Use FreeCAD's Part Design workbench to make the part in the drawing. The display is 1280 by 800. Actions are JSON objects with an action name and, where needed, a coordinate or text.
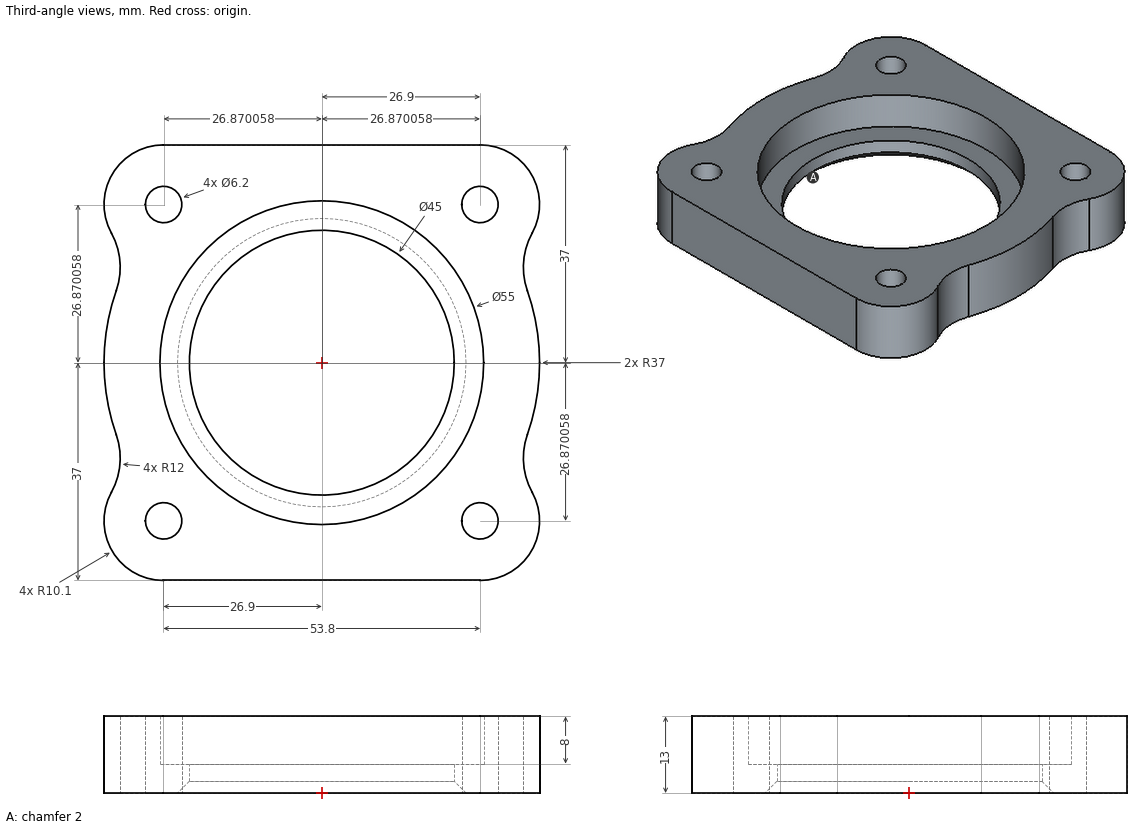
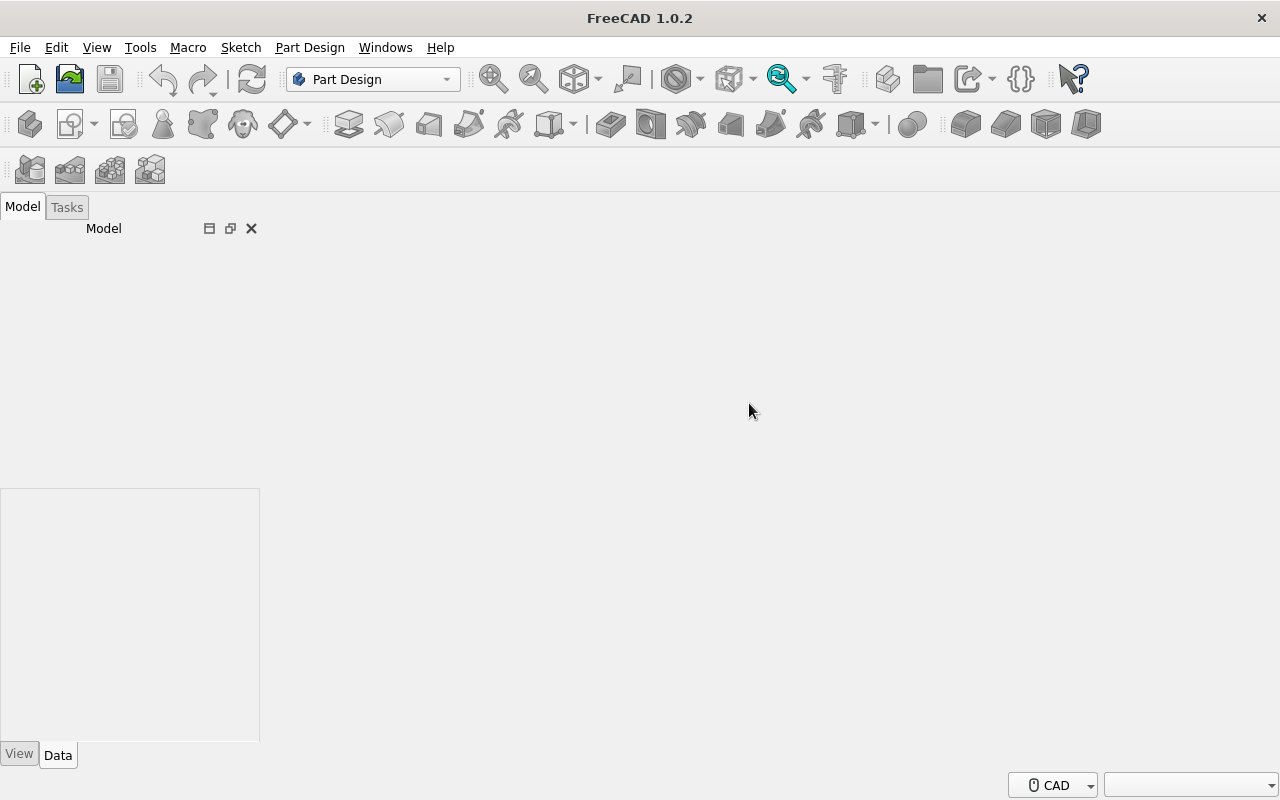
{"action": "key", "text": "ctrl+n"}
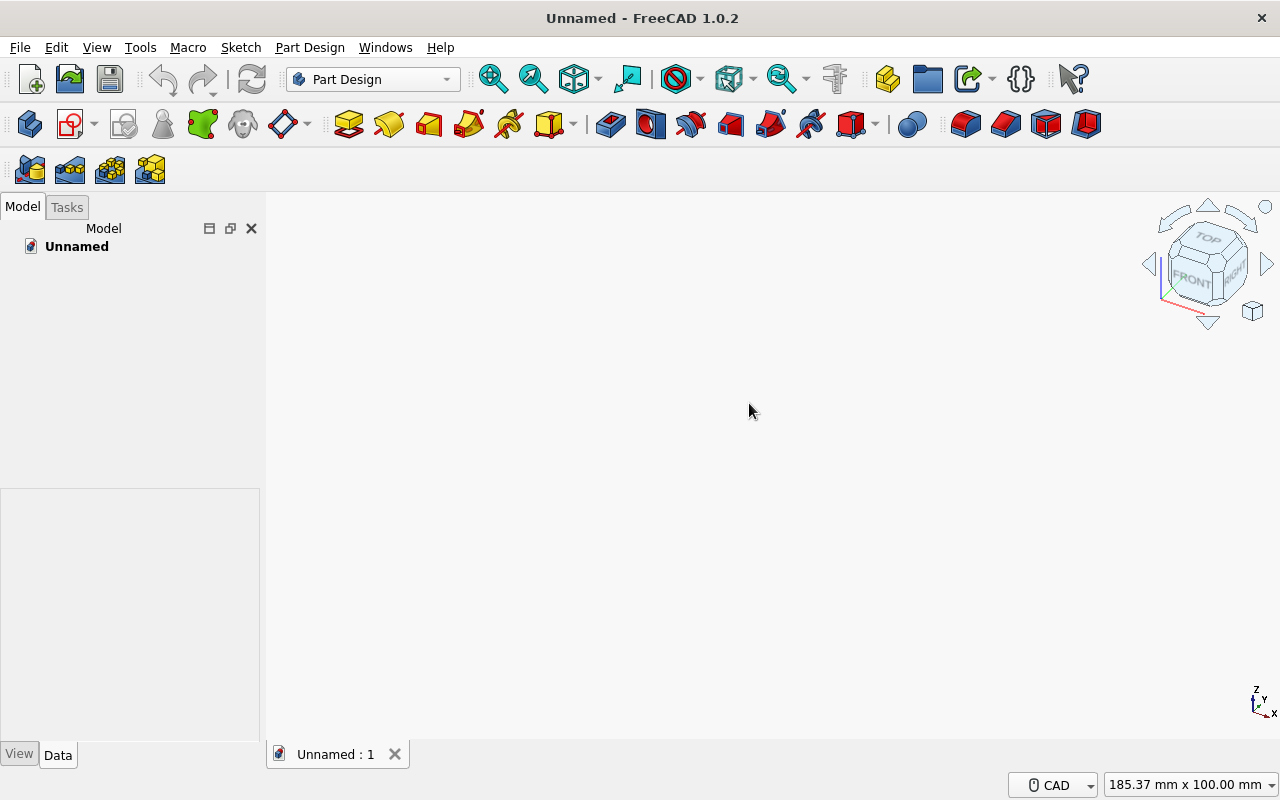
{"action": "left_click", "coordinate": [70, 124]}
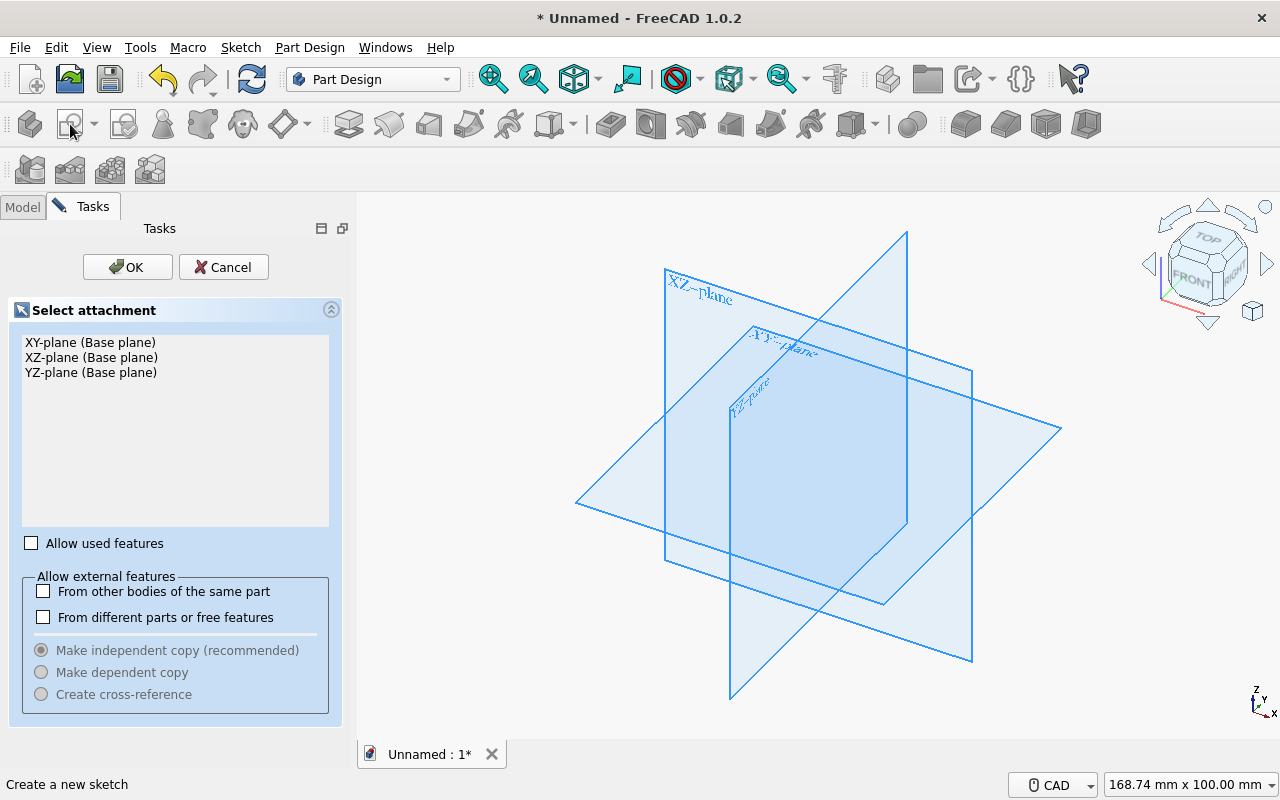
{"action": "left_click", "coordinate": [82, 342]}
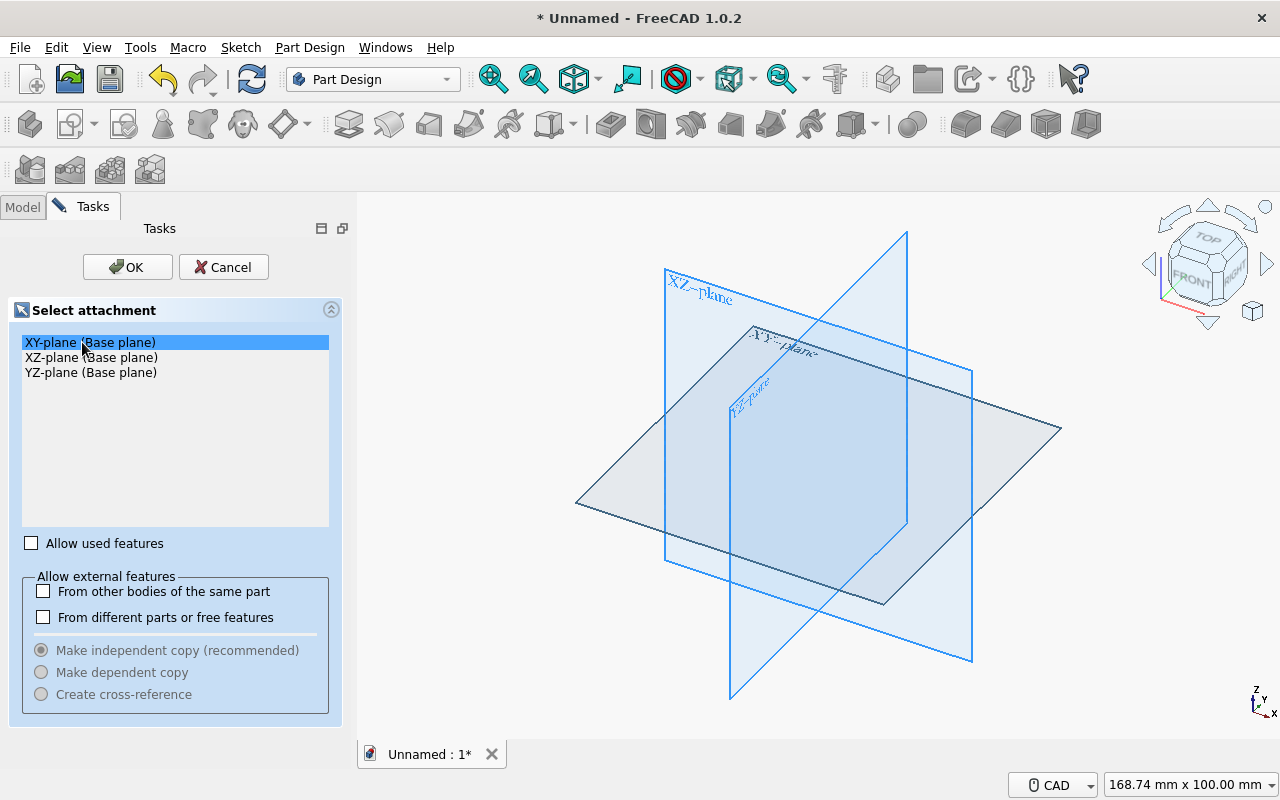
{"action": "left_click", "coordinate": [128, 267]}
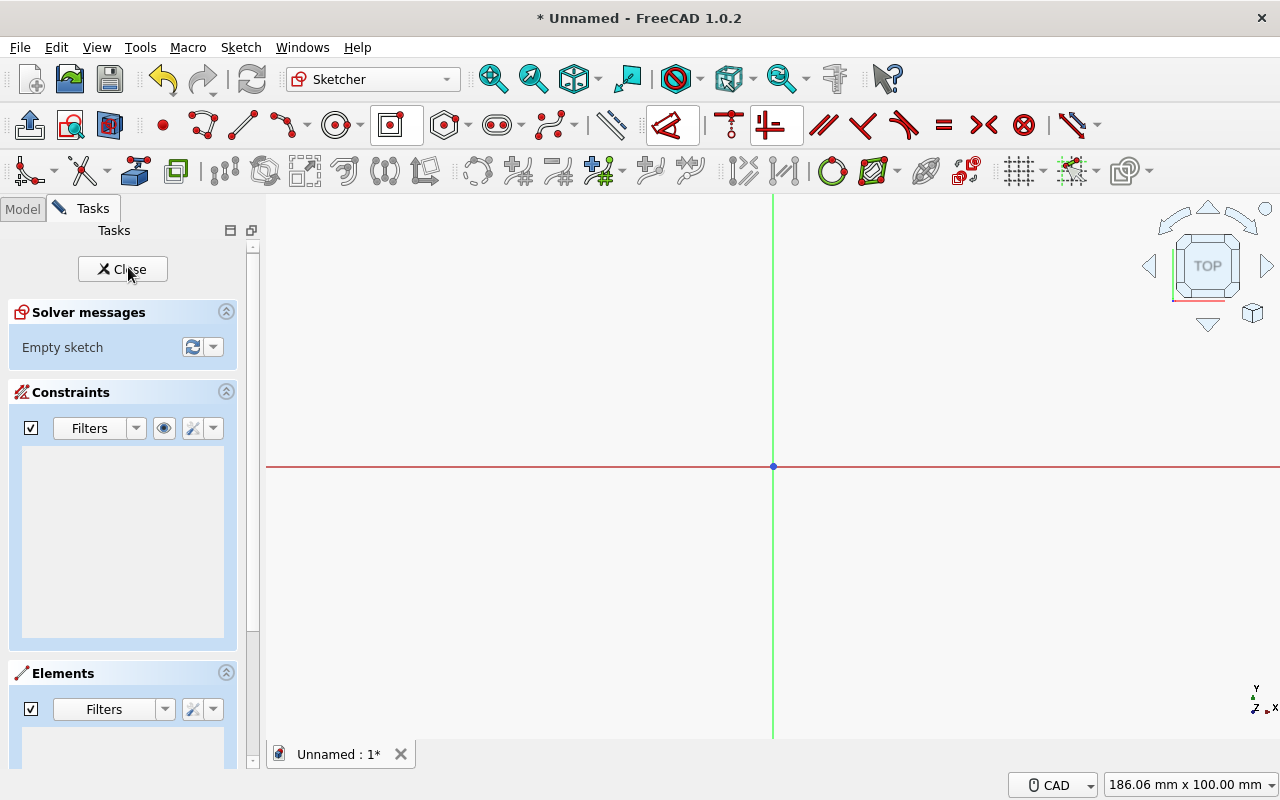
{"action": "left_click", "coordinate": [244, 126]}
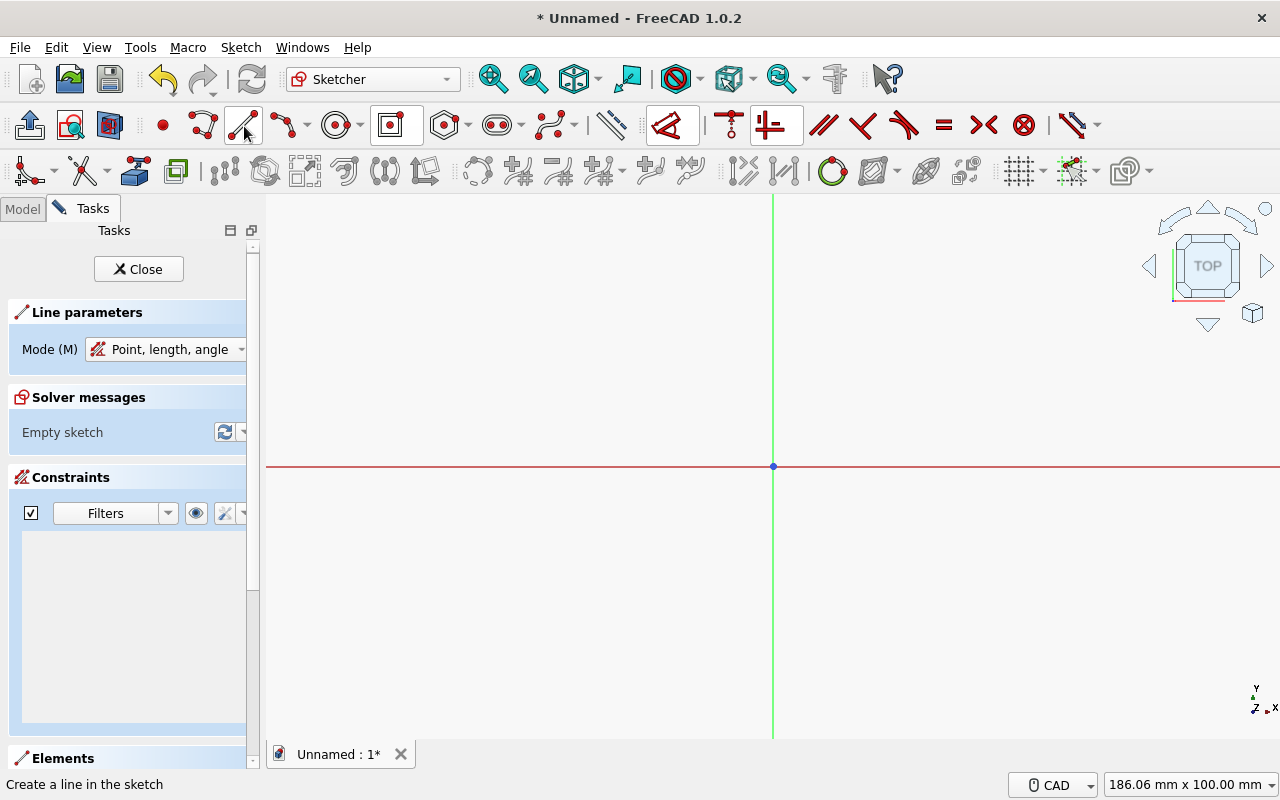
{"action": "left_click", "coordinate": [626, 668]}
{"action": "left_click", "coordinate": [920, 668]}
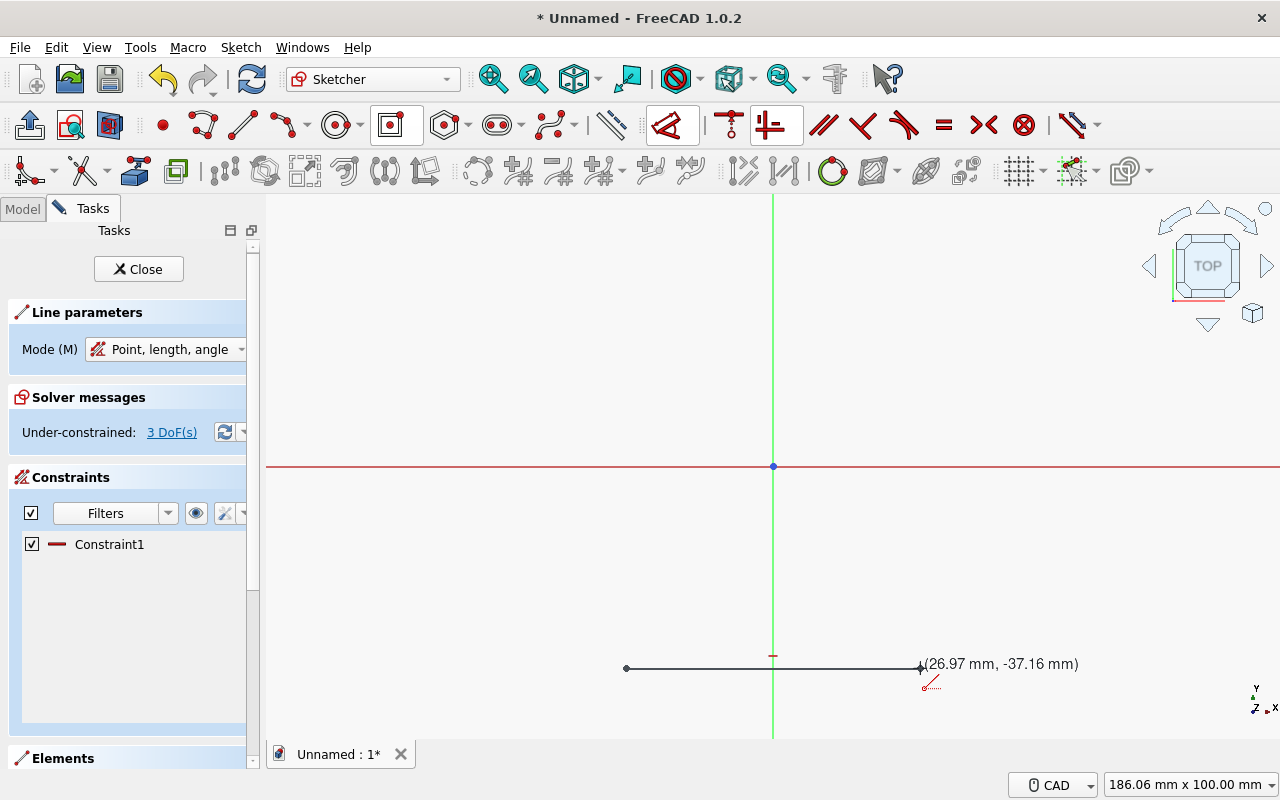
{"action": "left_click", "coordinate": [920, 265]}
{"action": "left_click", "coordinate": [626, 265]}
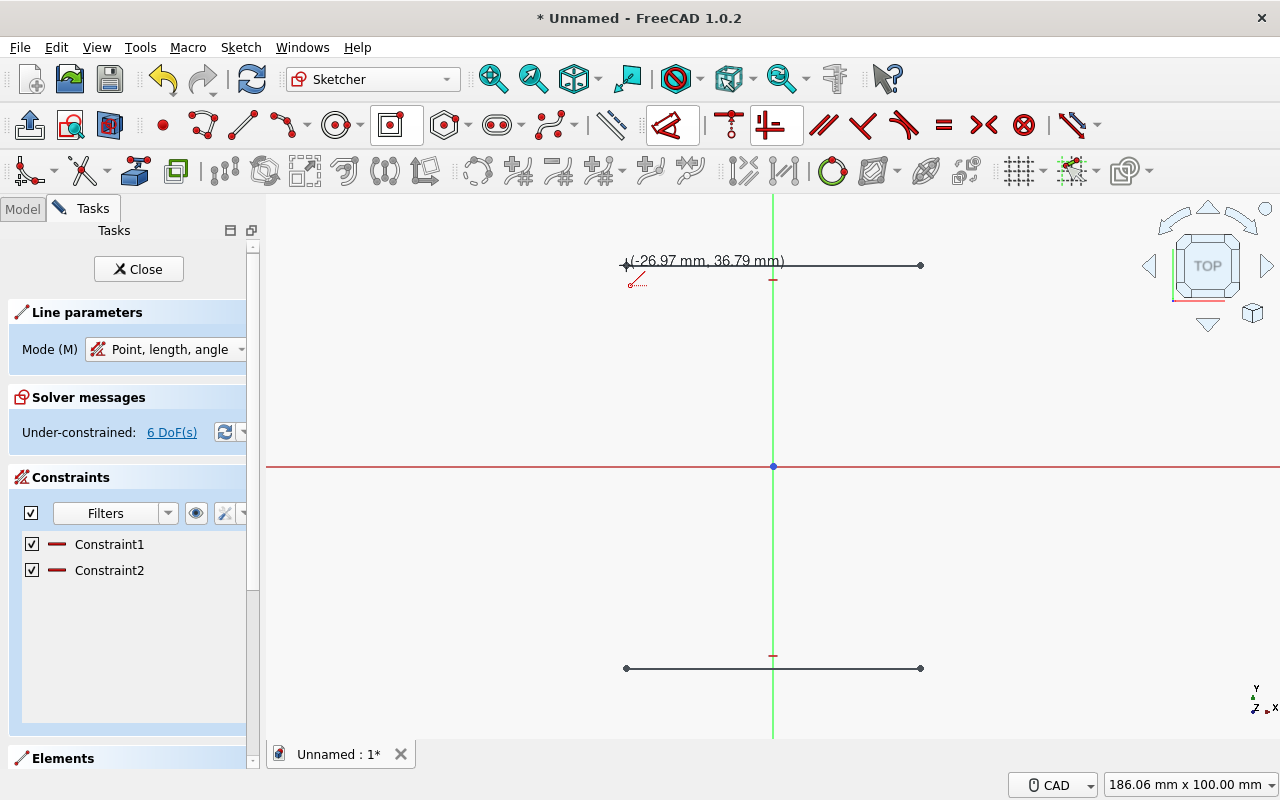
{"action": "key", "text": "g 3 a"}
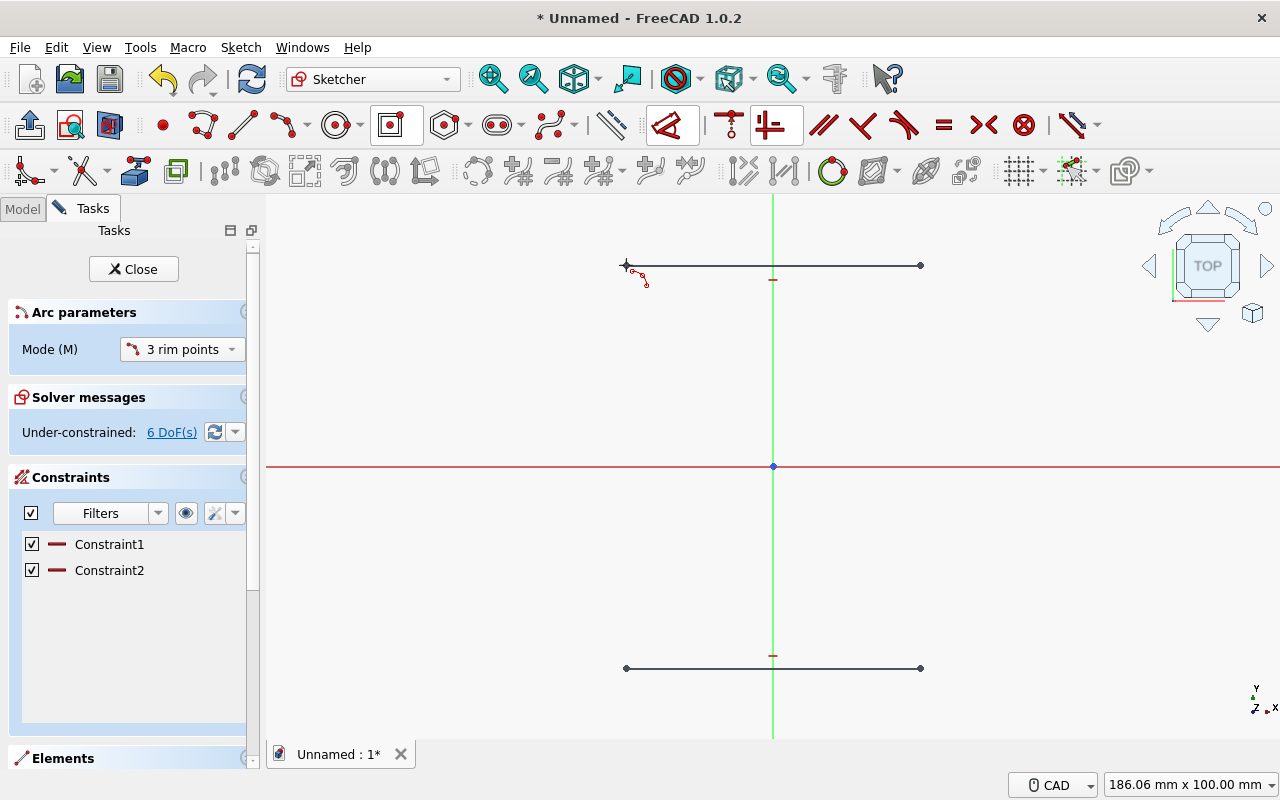
{"action": "left_click", "coordinate": [920, 669]}
{"action": "left_click", "coordinate": [968, 586]}
{"action": "left_click", "coordinate": [967, 641]}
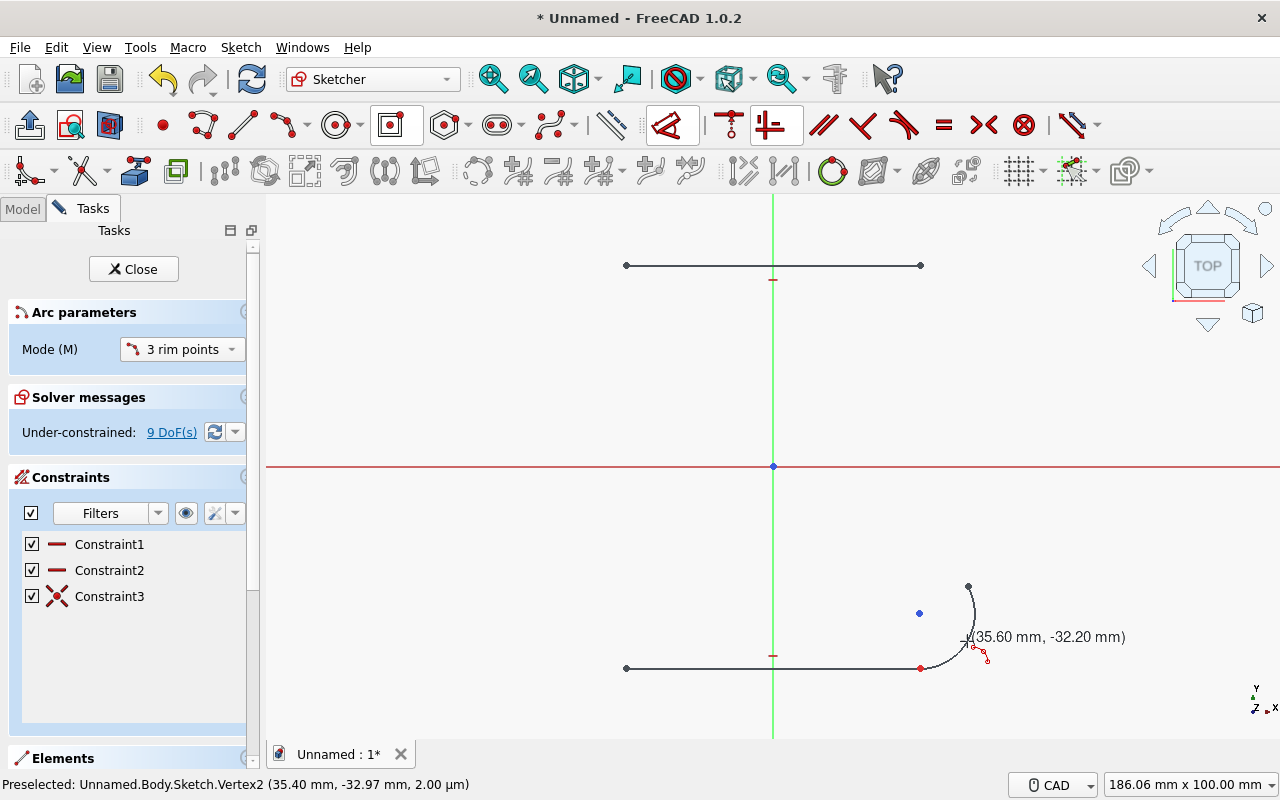
{"action": "left_click", "coordinate": [968, 587]}
{"action": "left_click", "coordinate": [963, 533]}